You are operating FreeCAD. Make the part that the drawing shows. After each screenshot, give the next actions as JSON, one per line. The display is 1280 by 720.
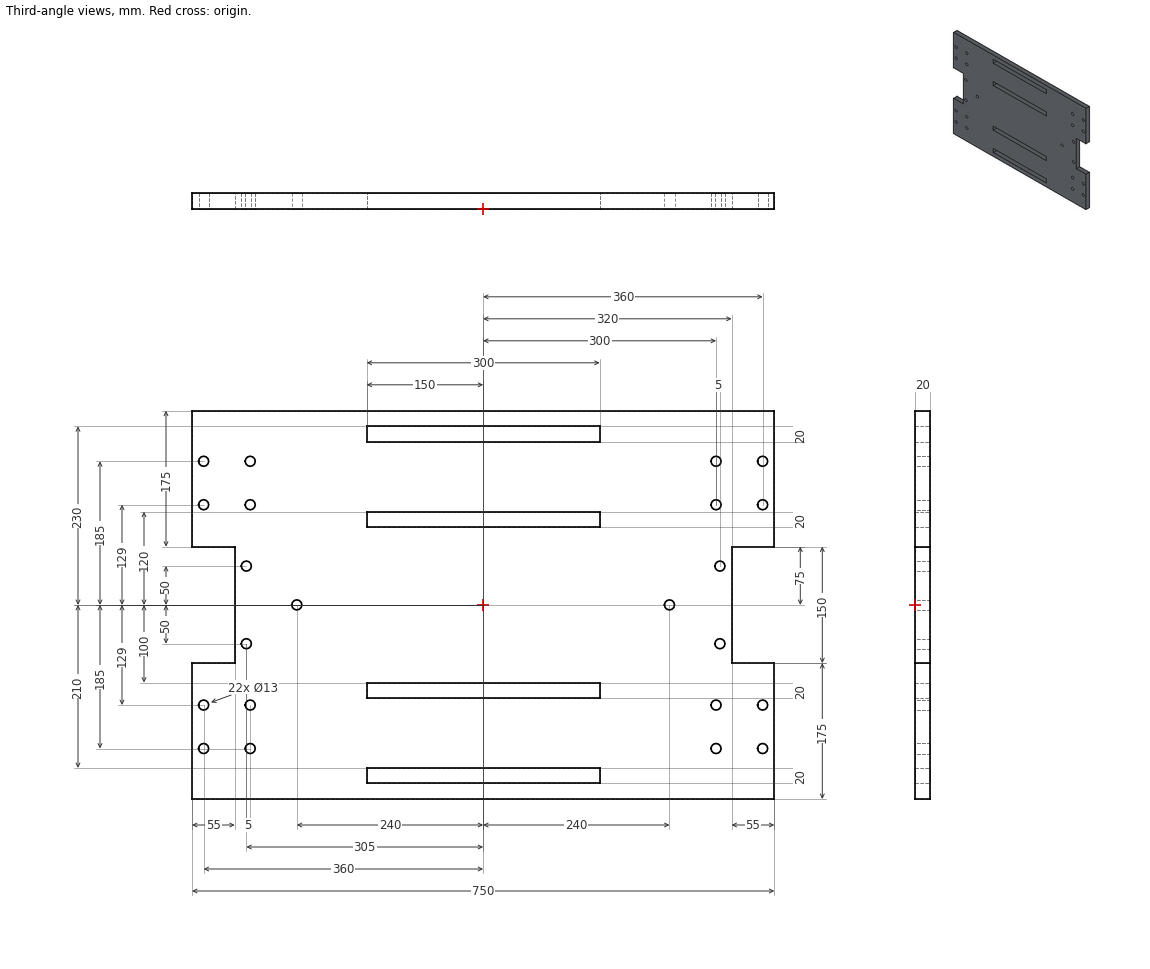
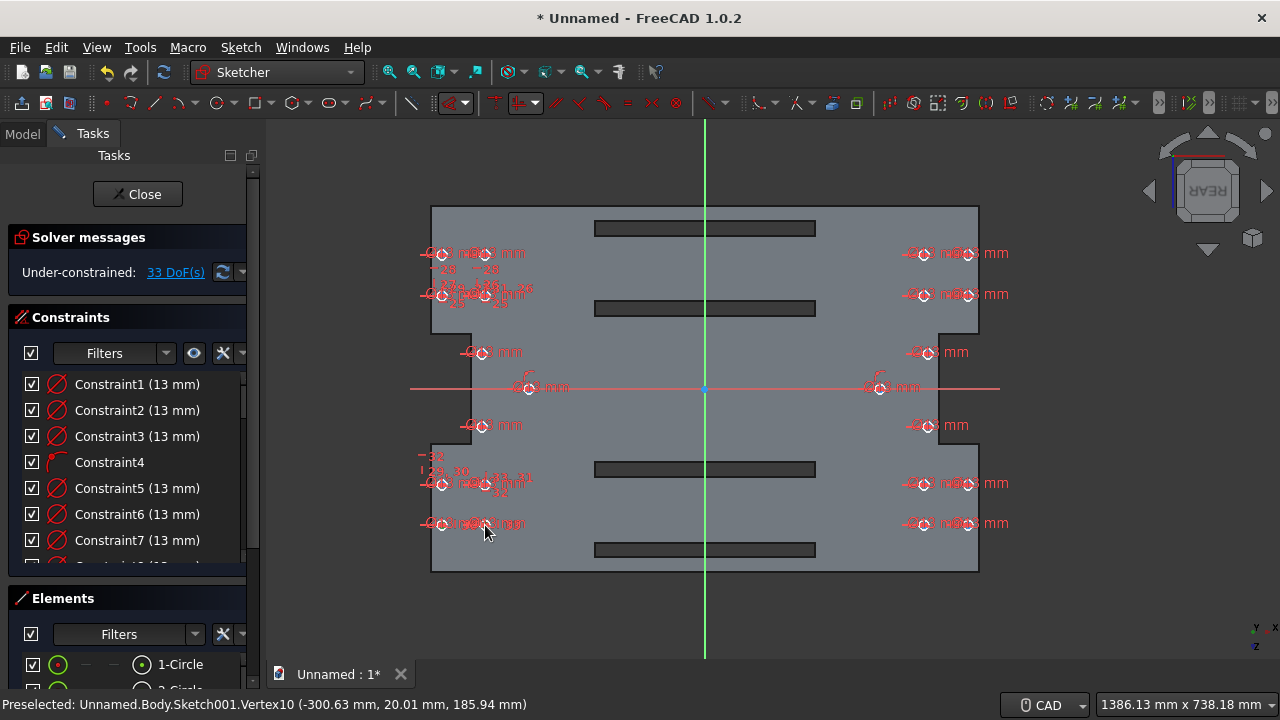
{"action": "key", "text": "h"}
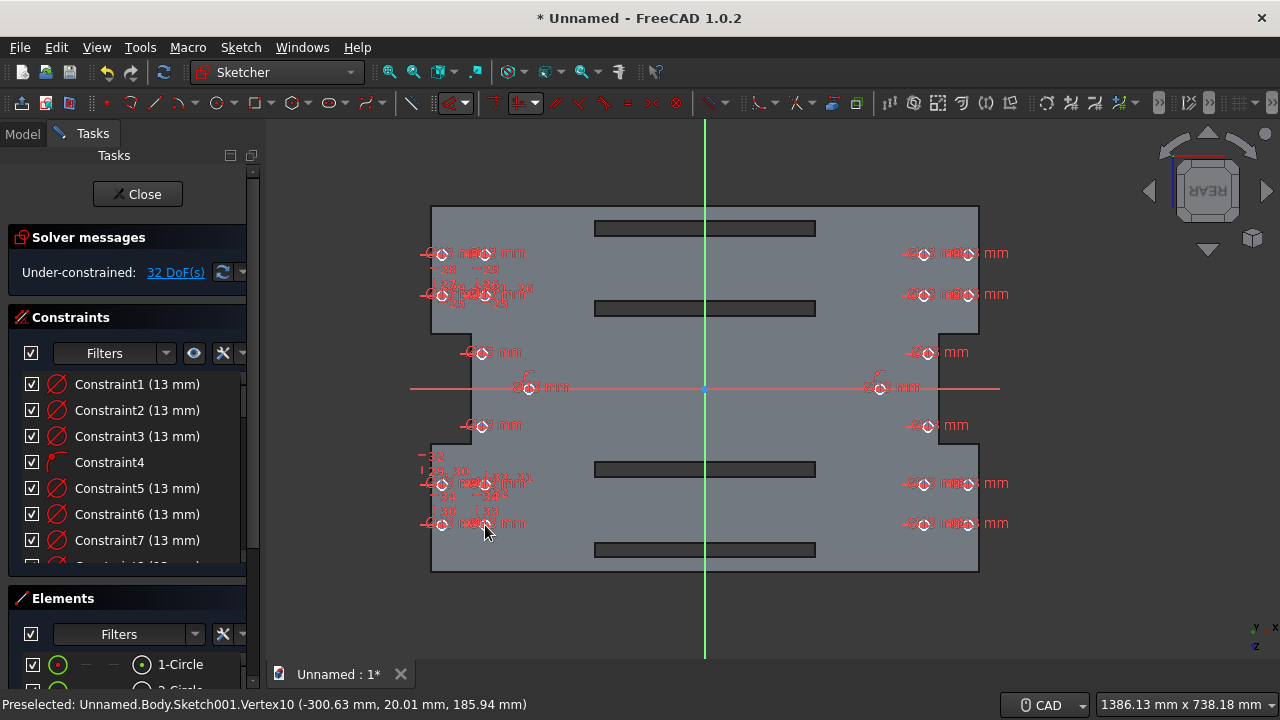
{"action": "left_click", "coordinate": [482, 354]}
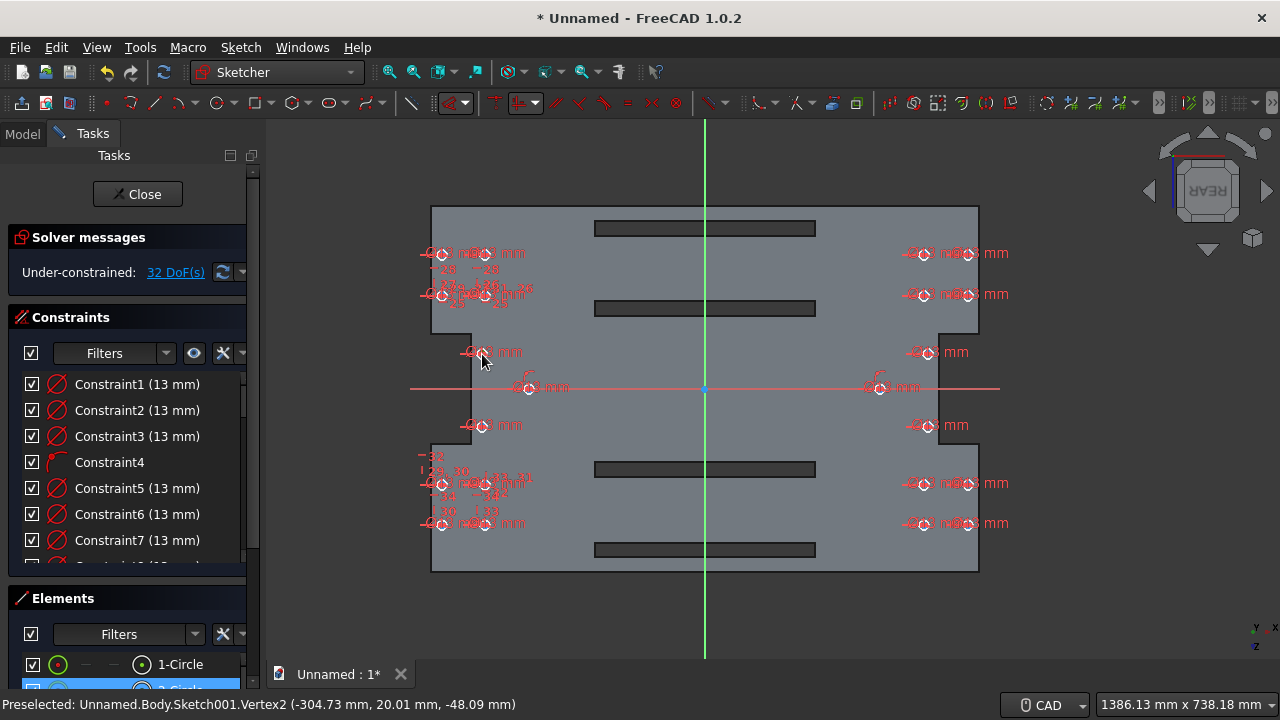
{"action": "left_click", "coordinate": [482, 427]}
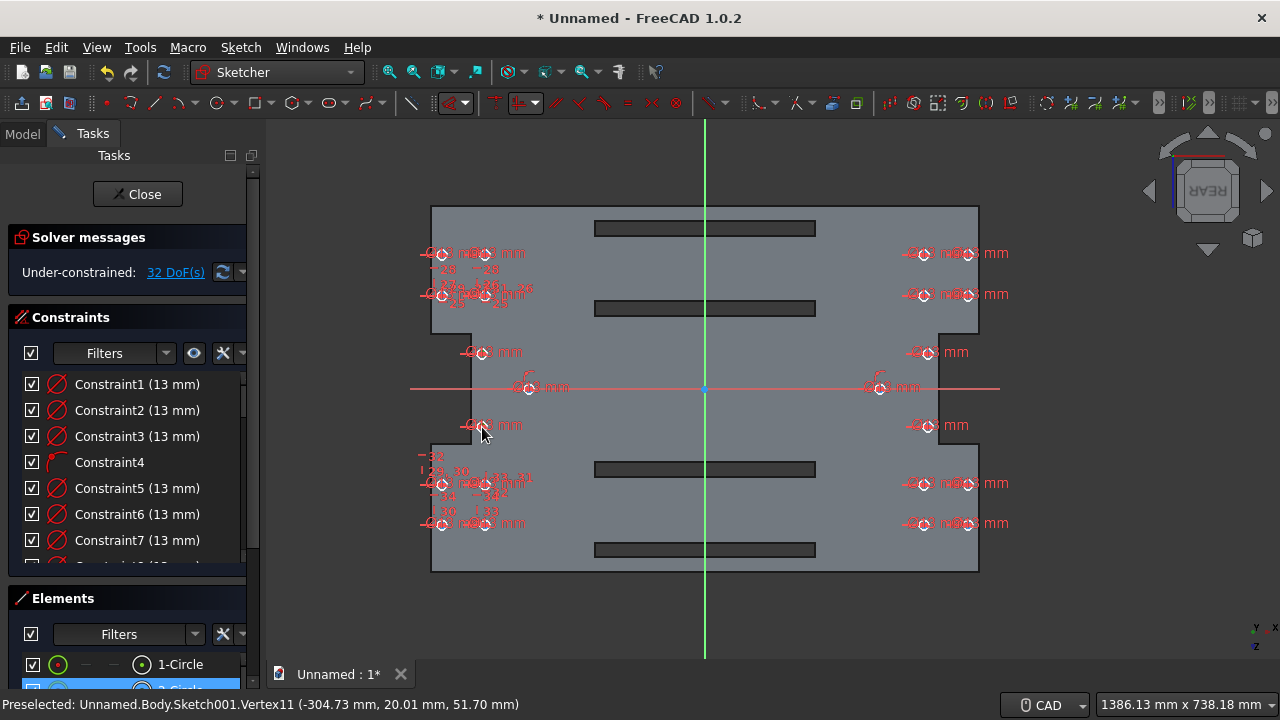
{"action": "key", "text": "v"}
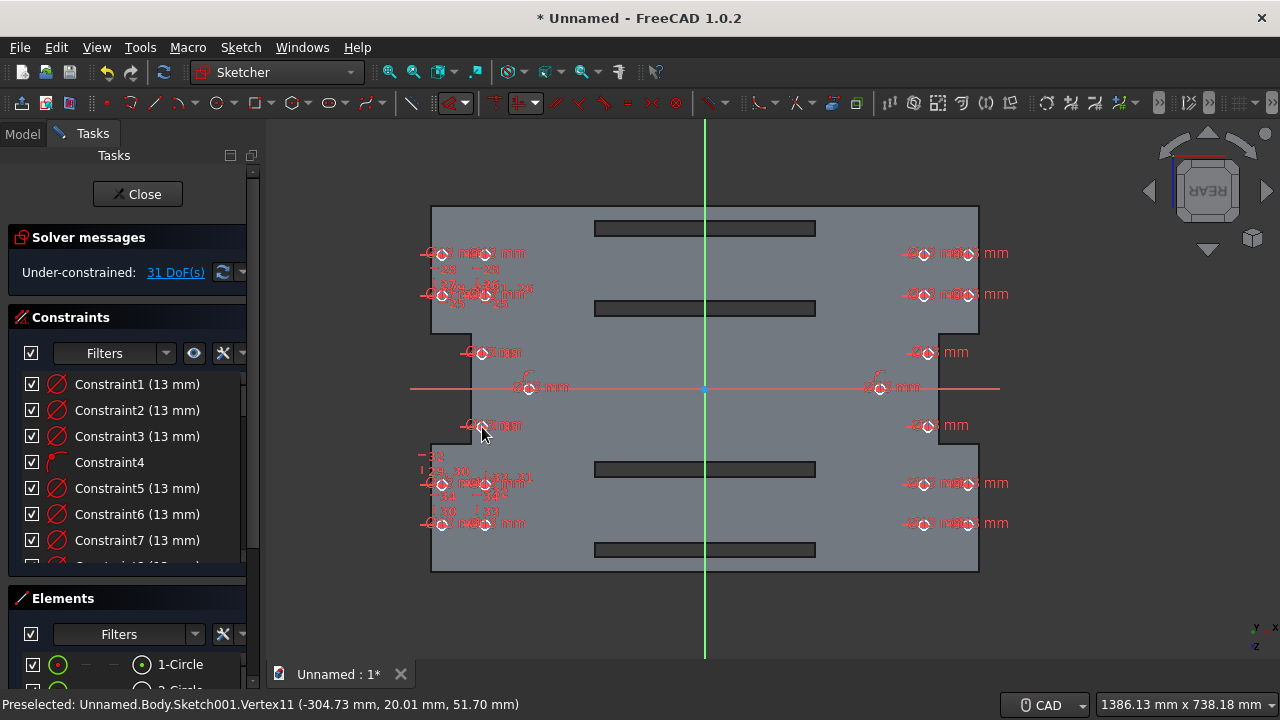
{"action": "left_click", "coordinate": [485, 485]}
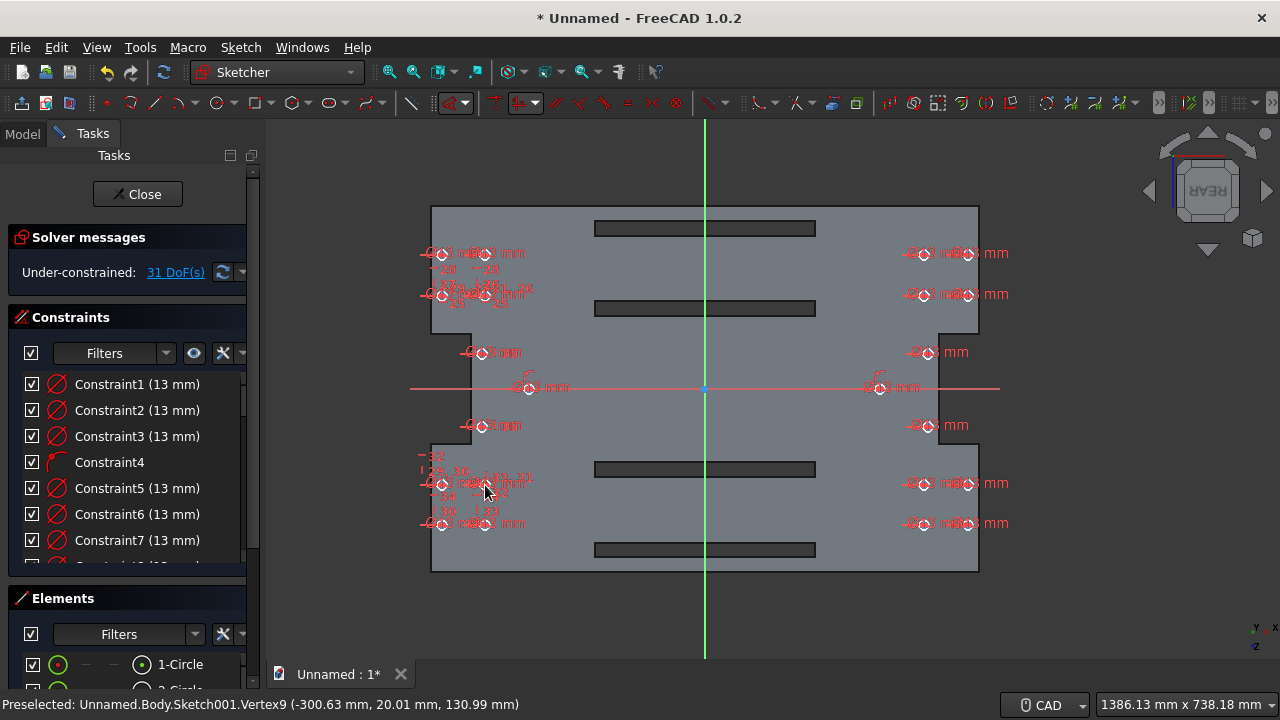
{"action": "left_click", "coordinate": [968, 485]}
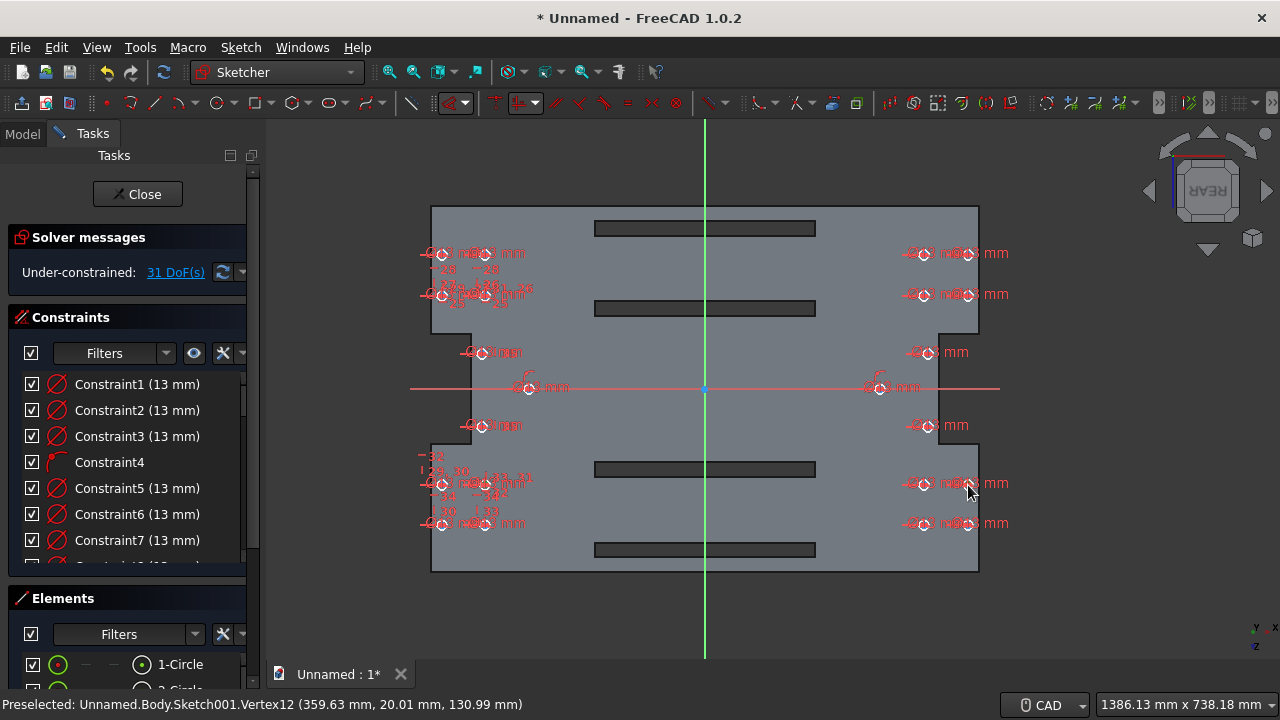
{"action": "key", "text": "h"}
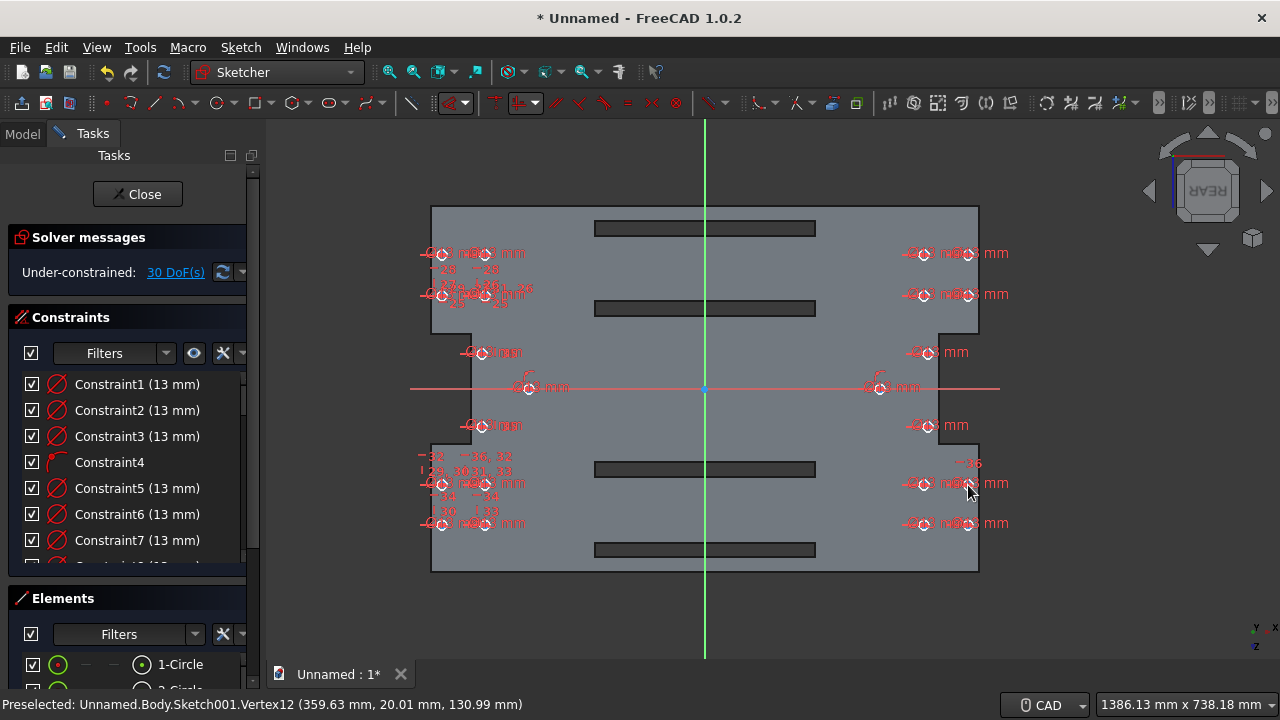
{"action": "left_click", "coordinate": [968, 485]}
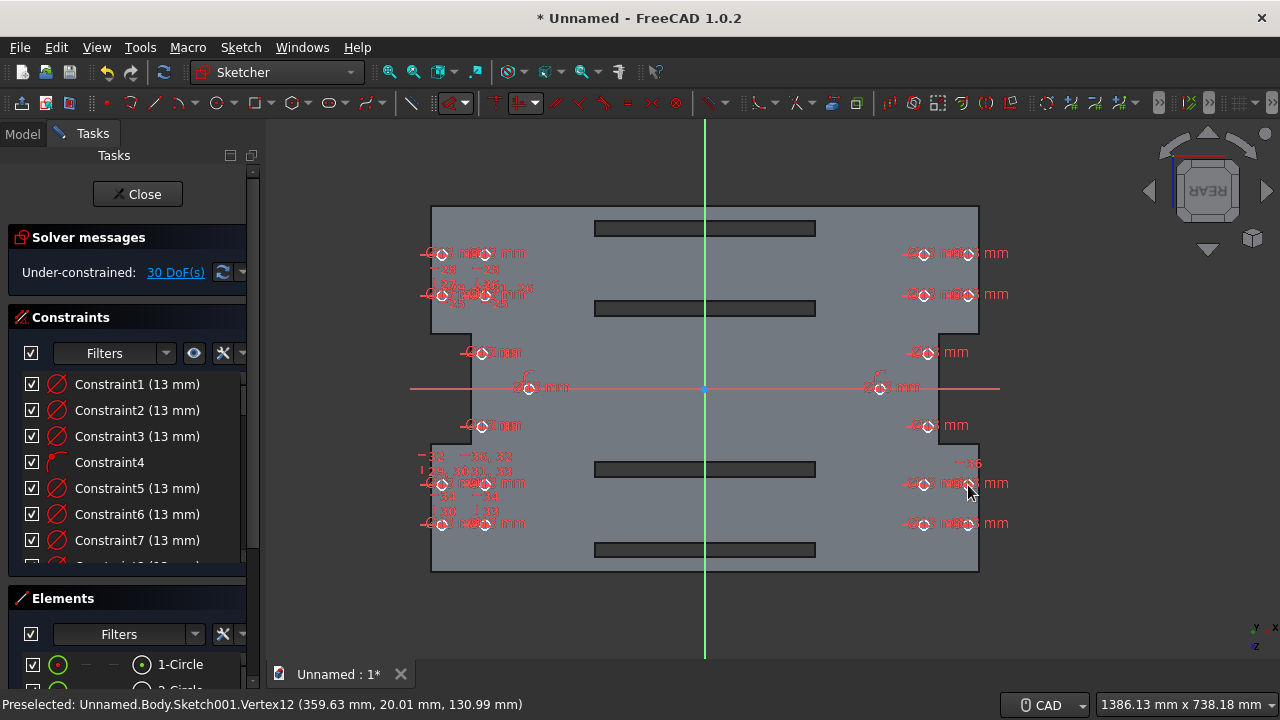
{"action": "left_click", "coordinate": [924, 485]}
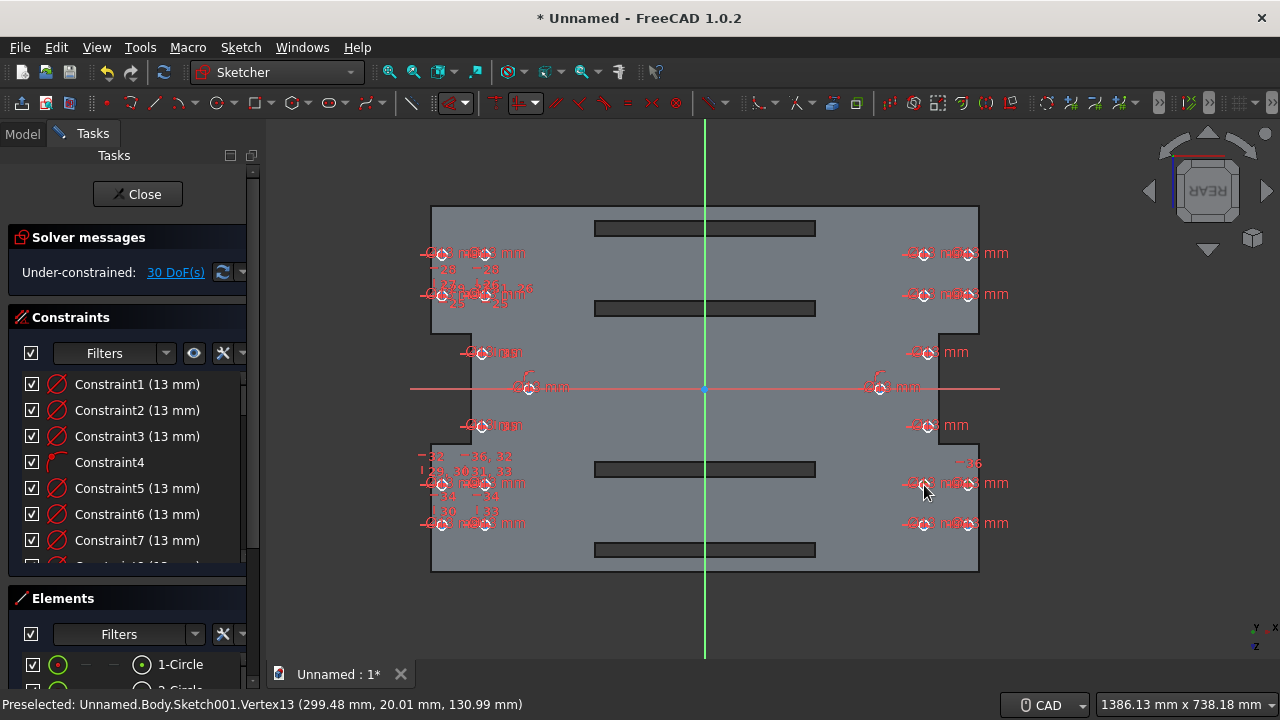
{"action": "left_click", "coordinate": [538, 104]}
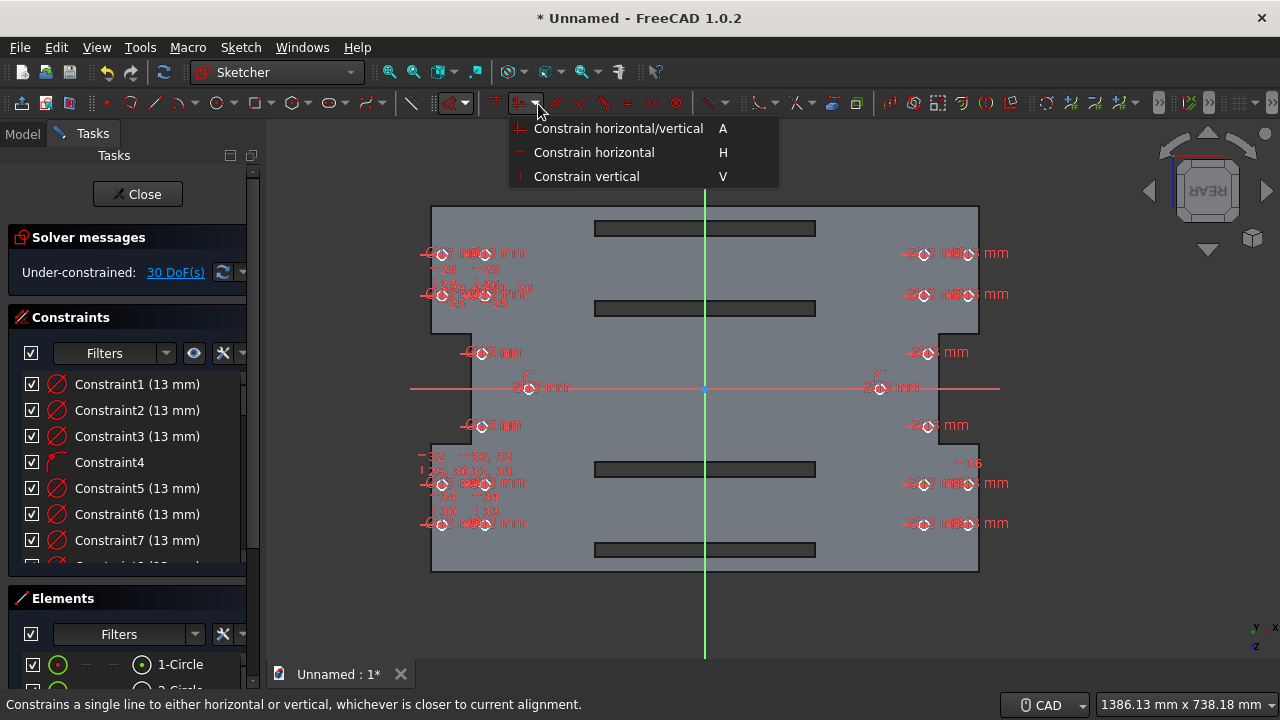
{"action": "left_click", "coordinate": [644, 152]}